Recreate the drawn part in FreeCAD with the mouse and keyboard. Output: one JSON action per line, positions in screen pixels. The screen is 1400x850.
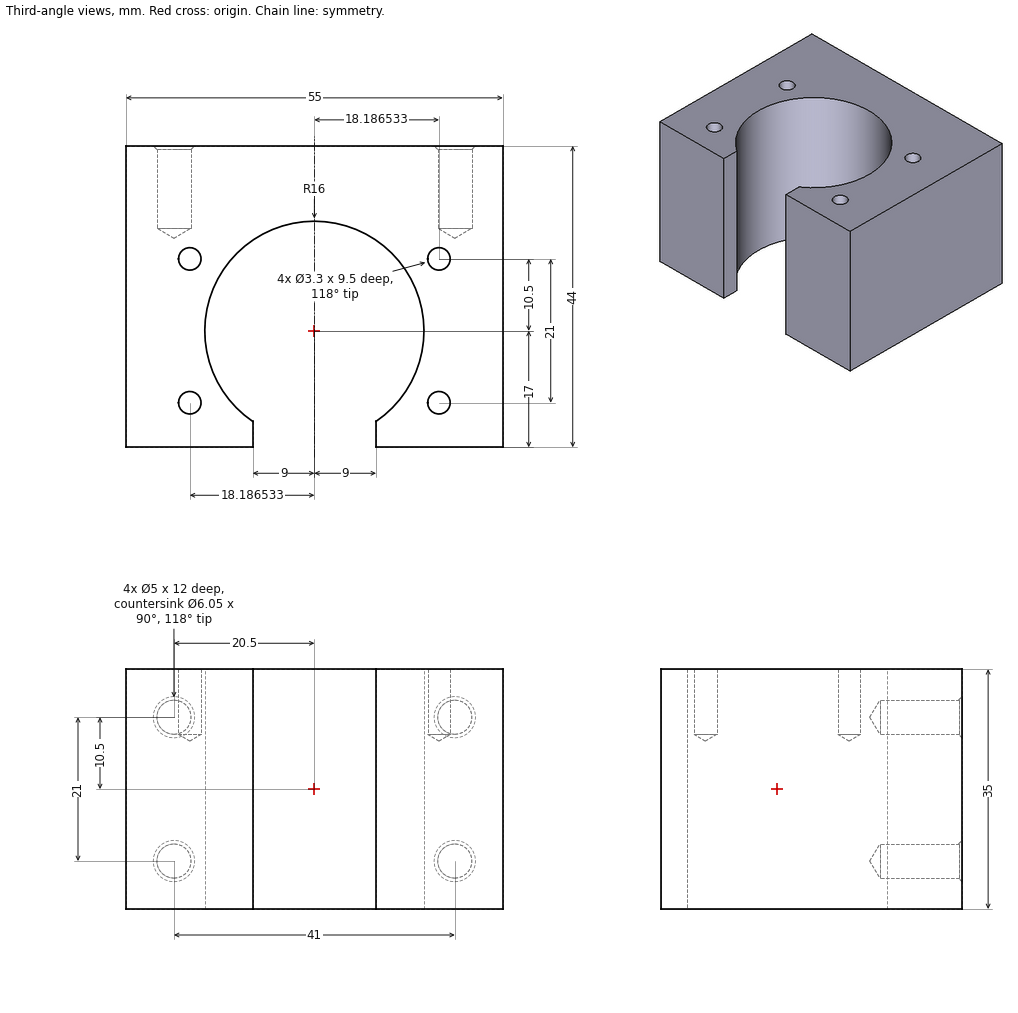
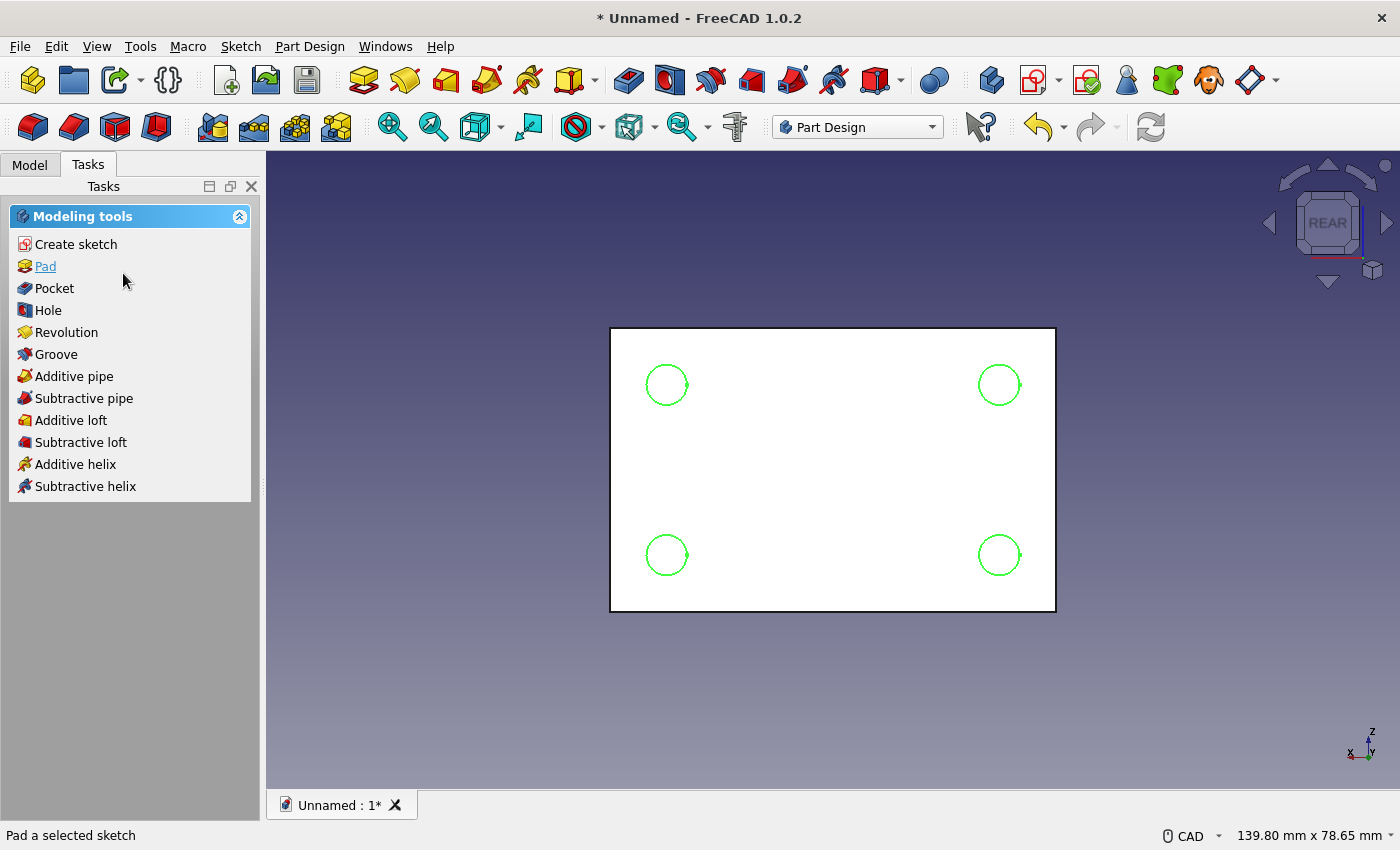
{"action": "left_click", "coordinate": [670, 80]}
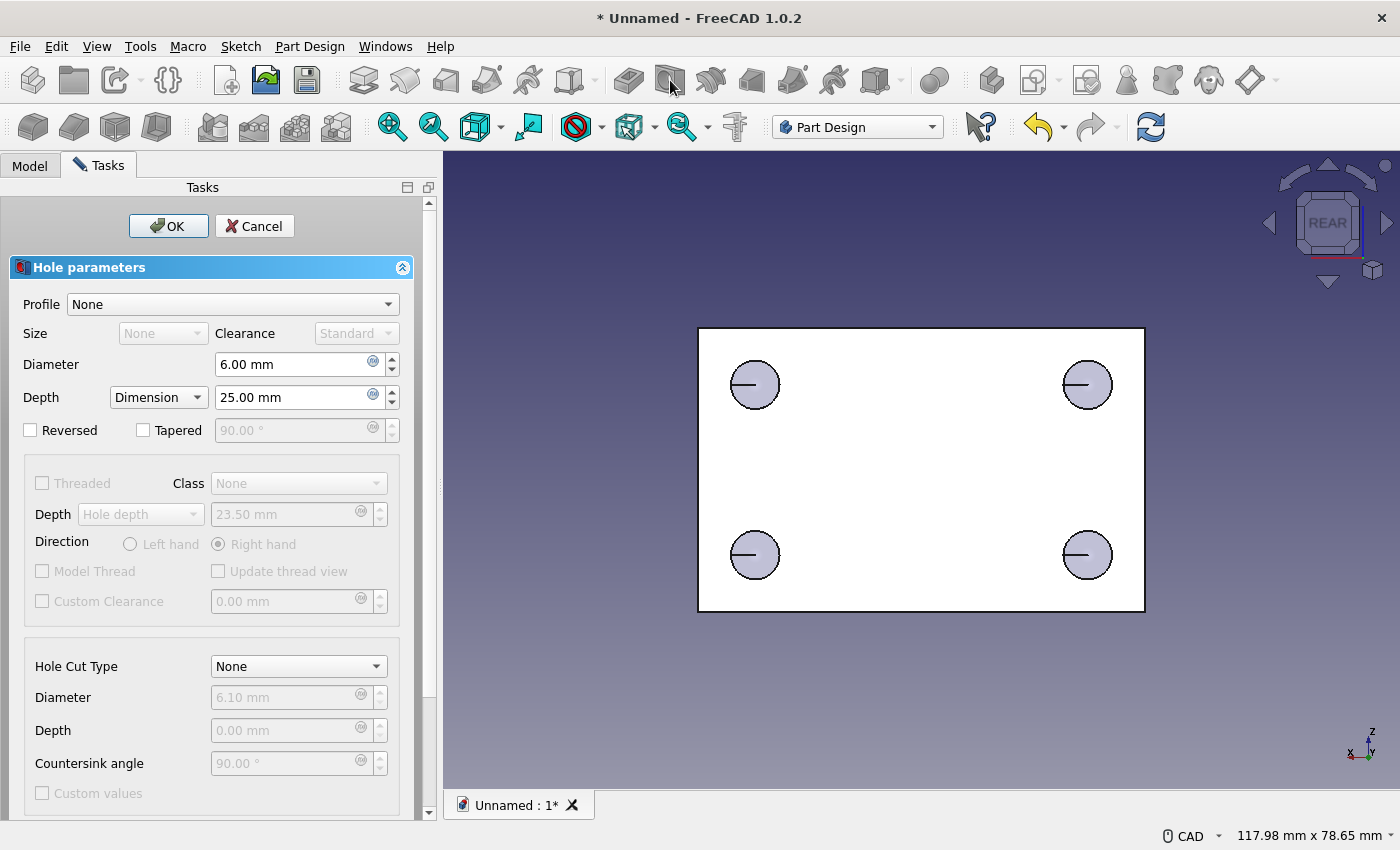
{"action": "triple_click", "coordinate": [300, 364]}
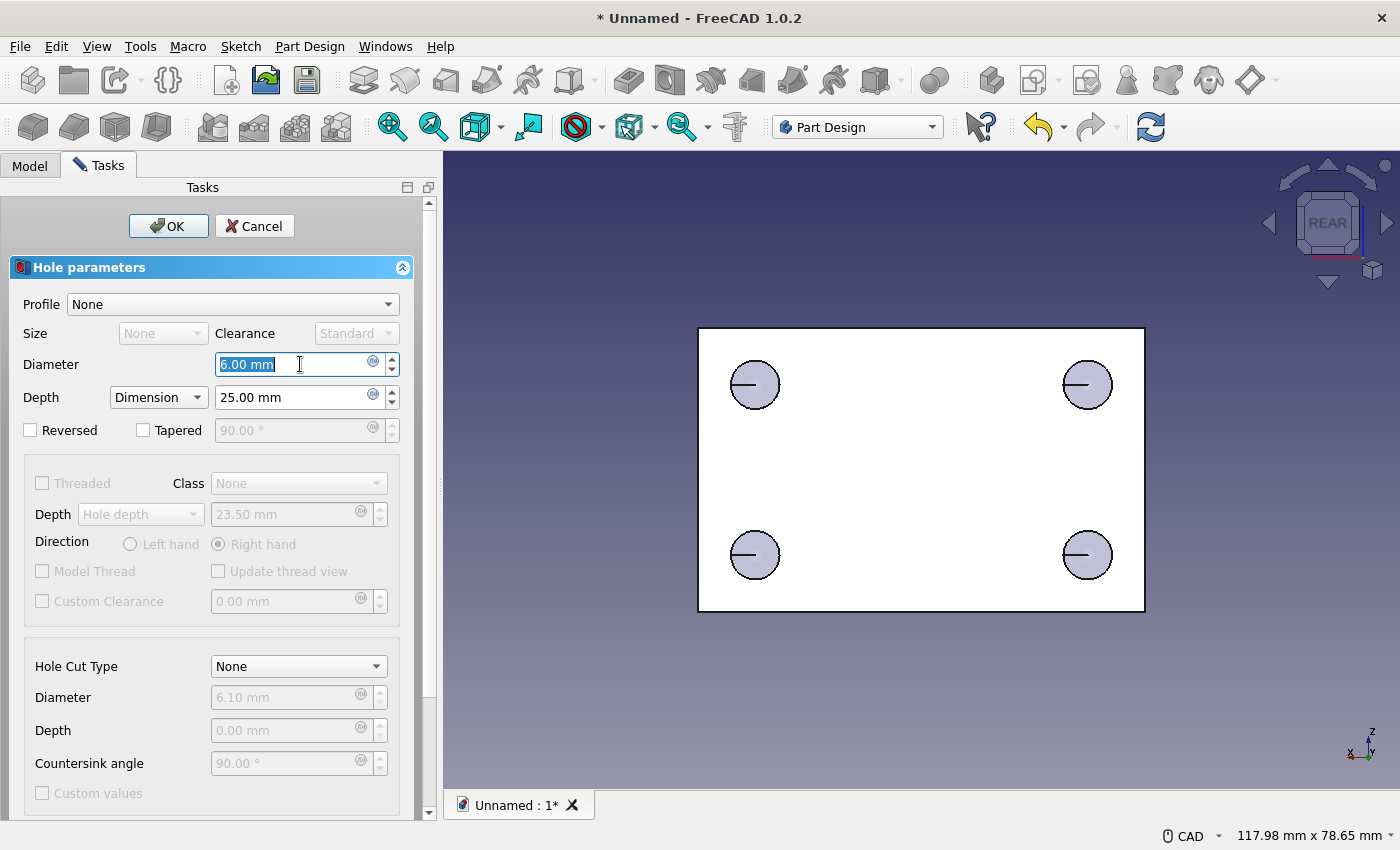
{"action": "type", "text": "5"}
{"action": "key", "text": "Tab"}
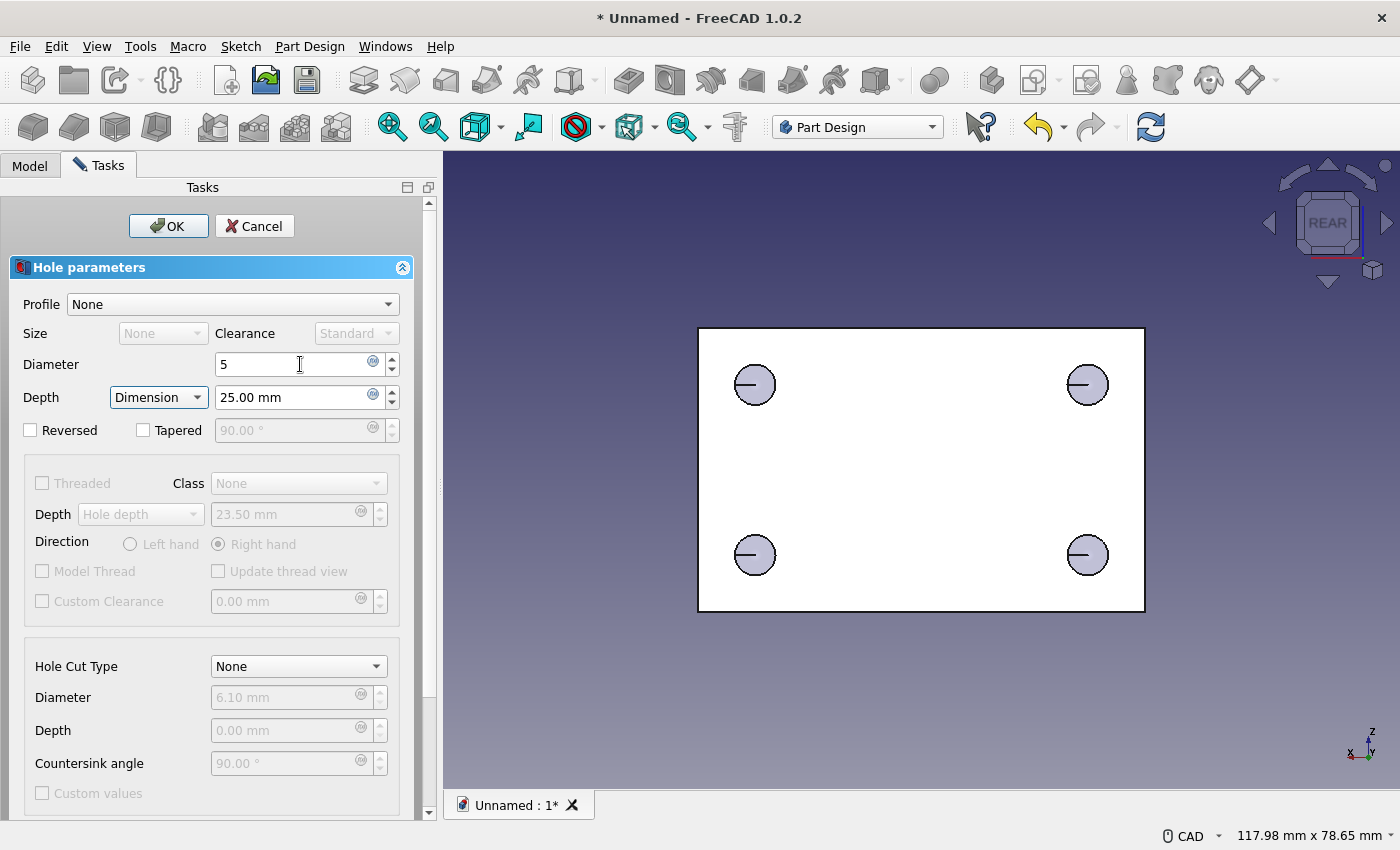
{"action": "triple_click", "coordinate": [300, 398]}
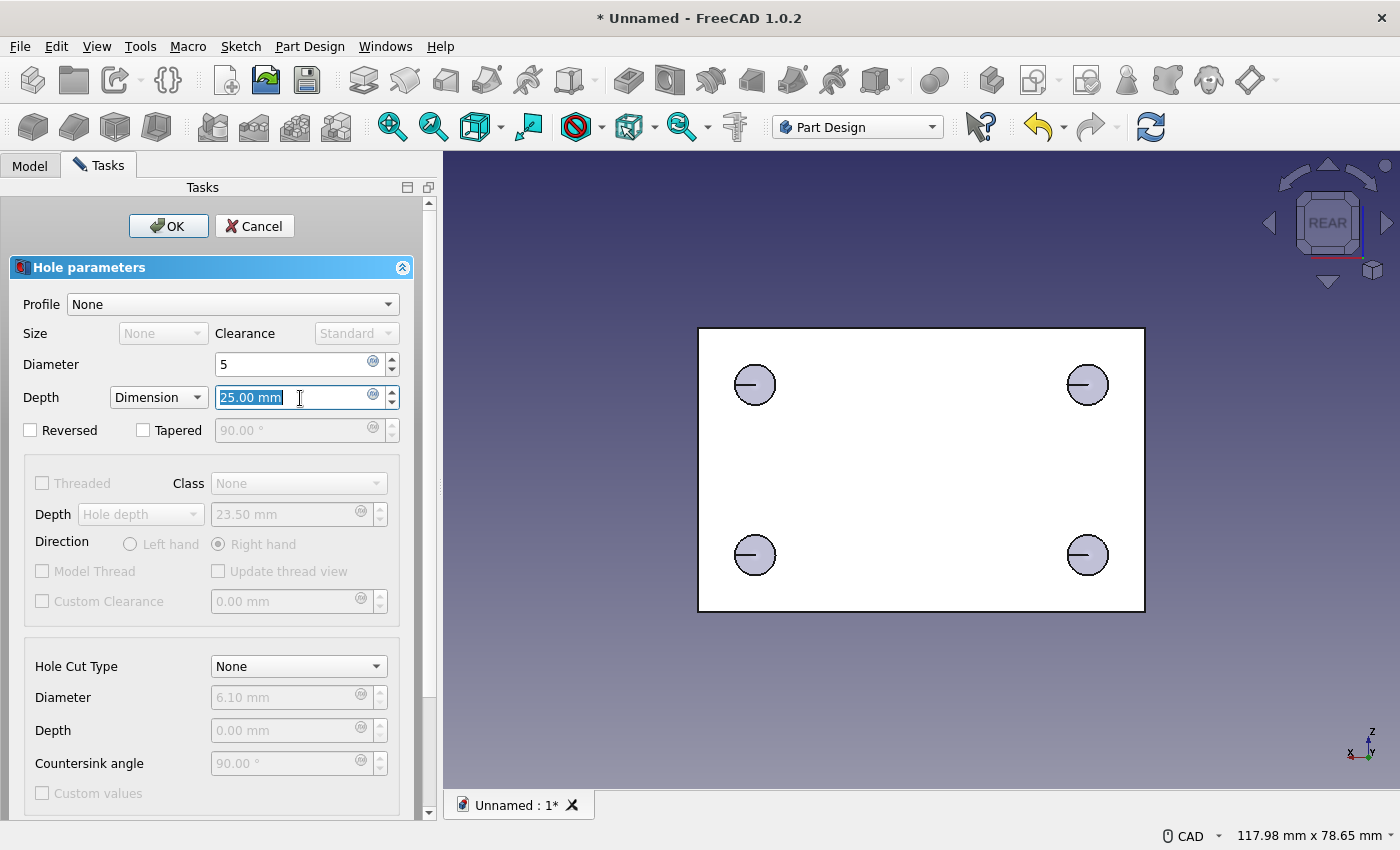
{"action": "type", "text": "12"}
{"action": "key", "text": "Tab"}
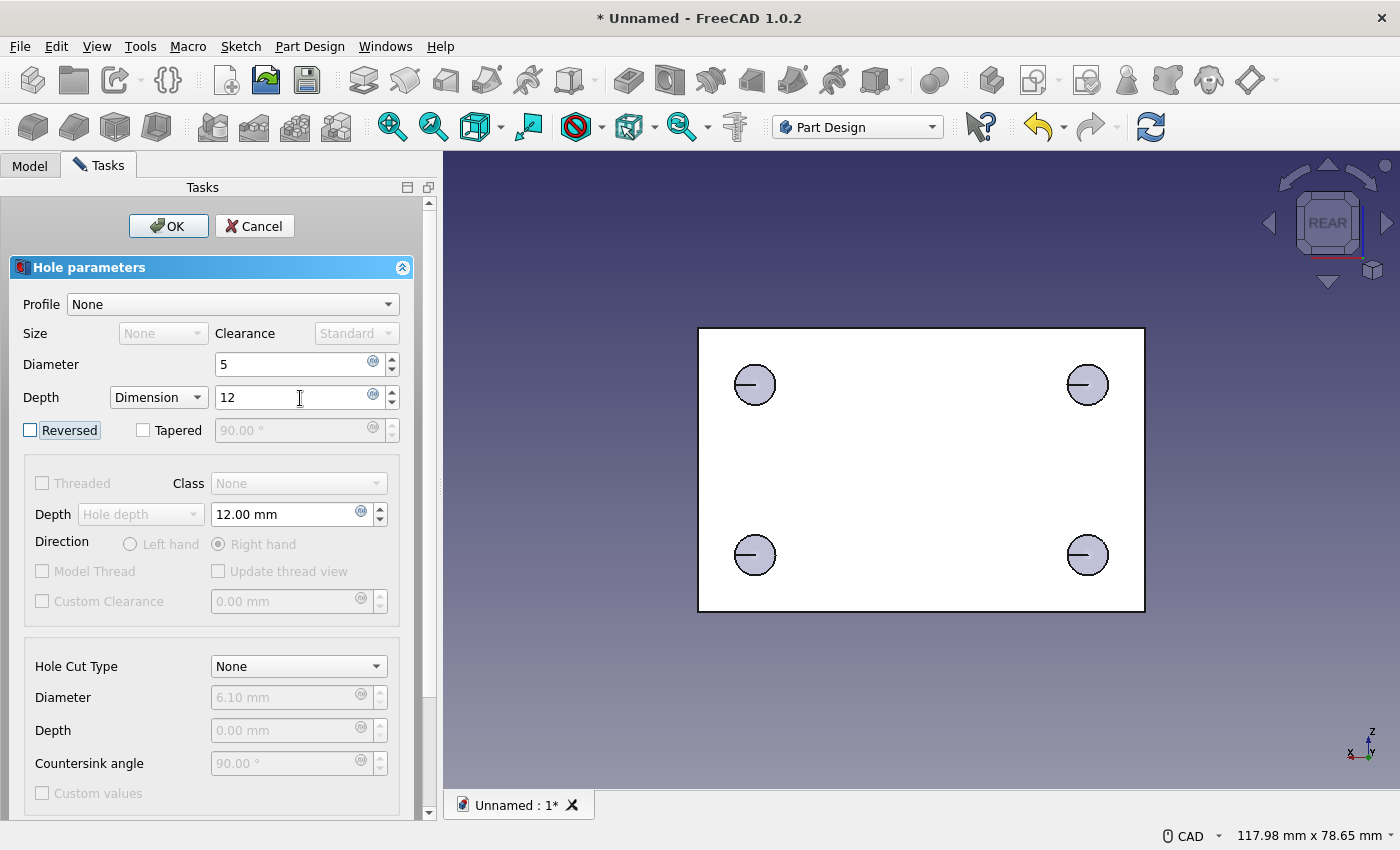
{"action": "left_click", "coordinate": [300, 666]}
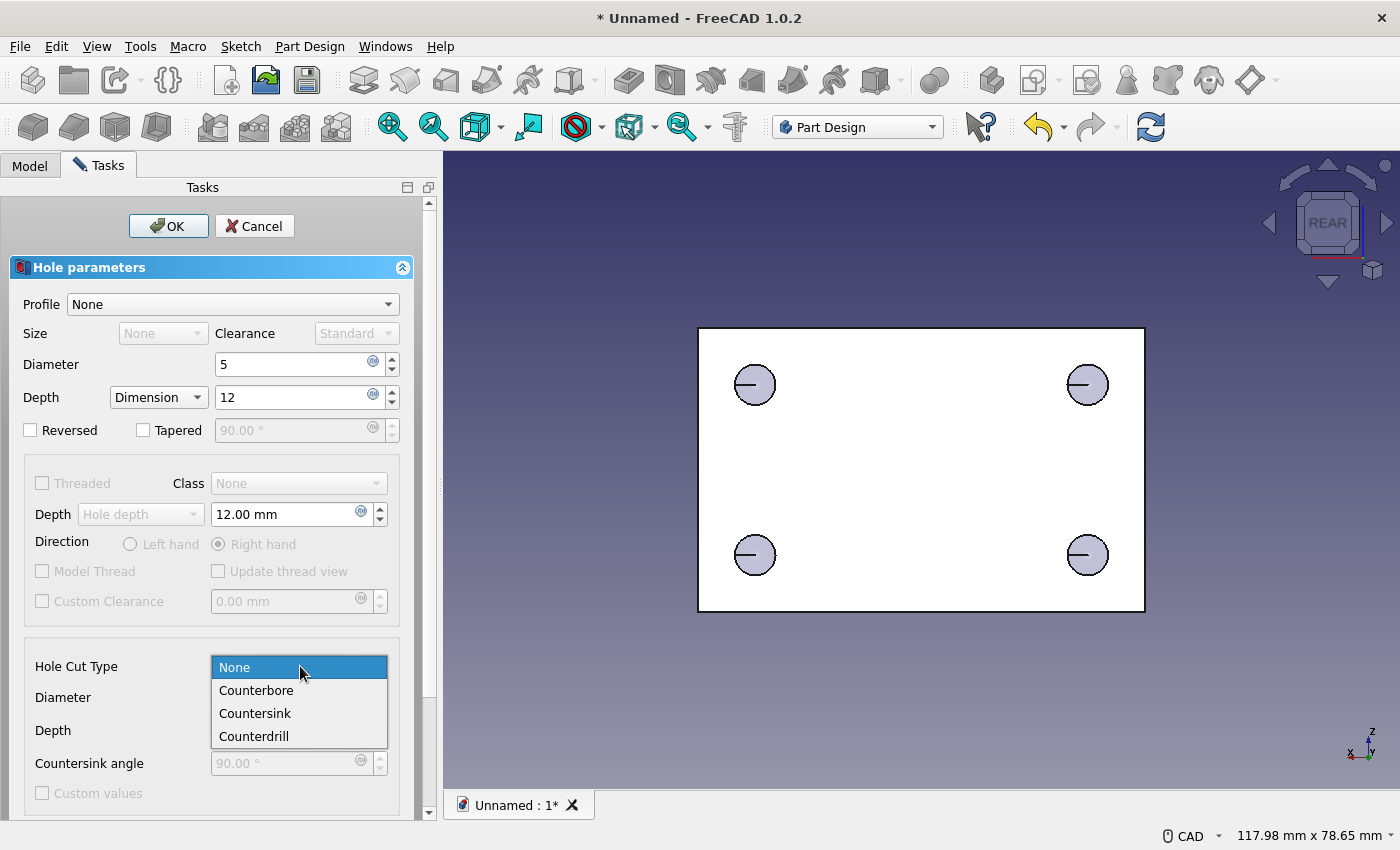
{"action": "left_click", "coordinate": [298, 714]}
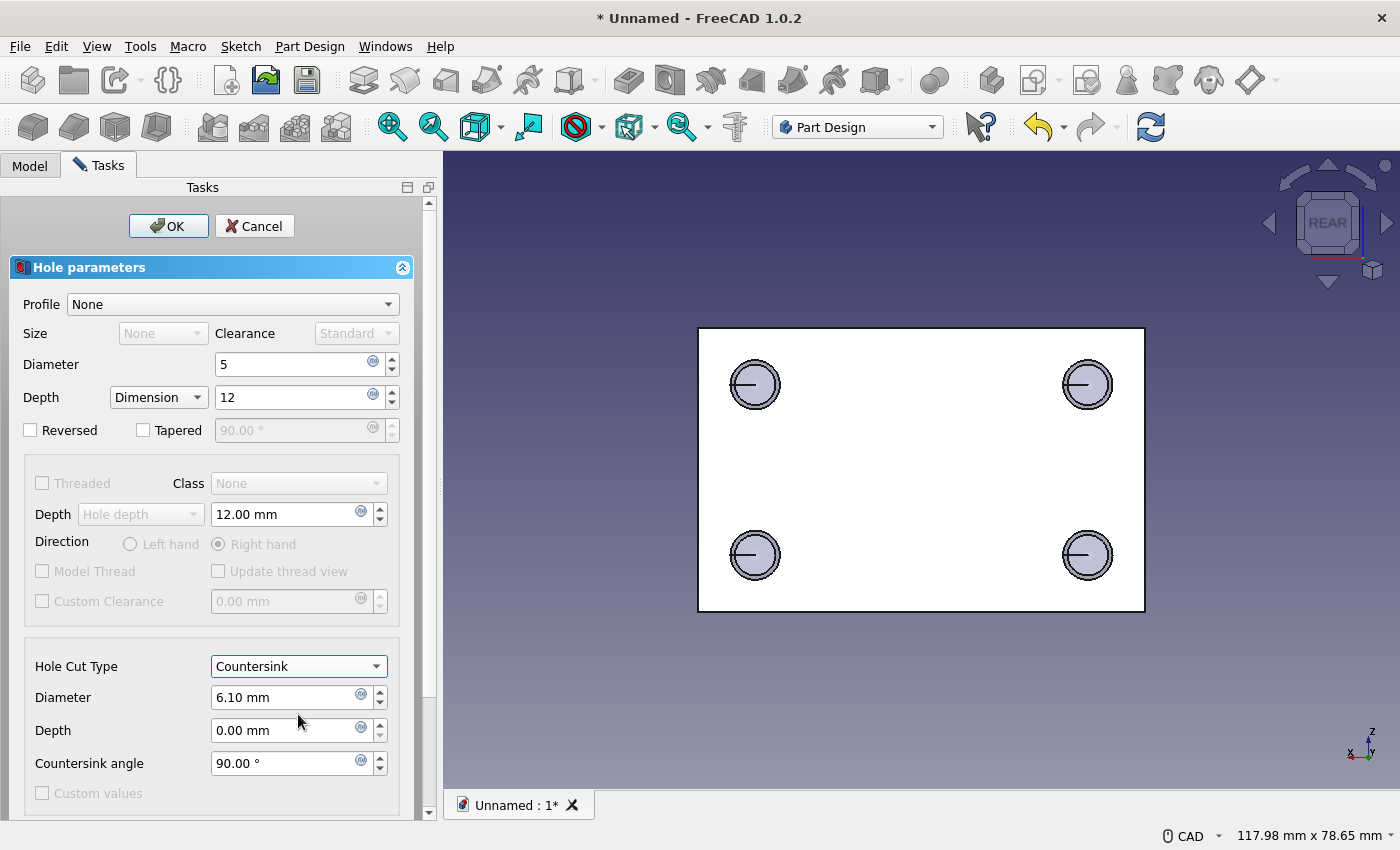
{"action": "triple_click", "coordinate": [292, 698]}